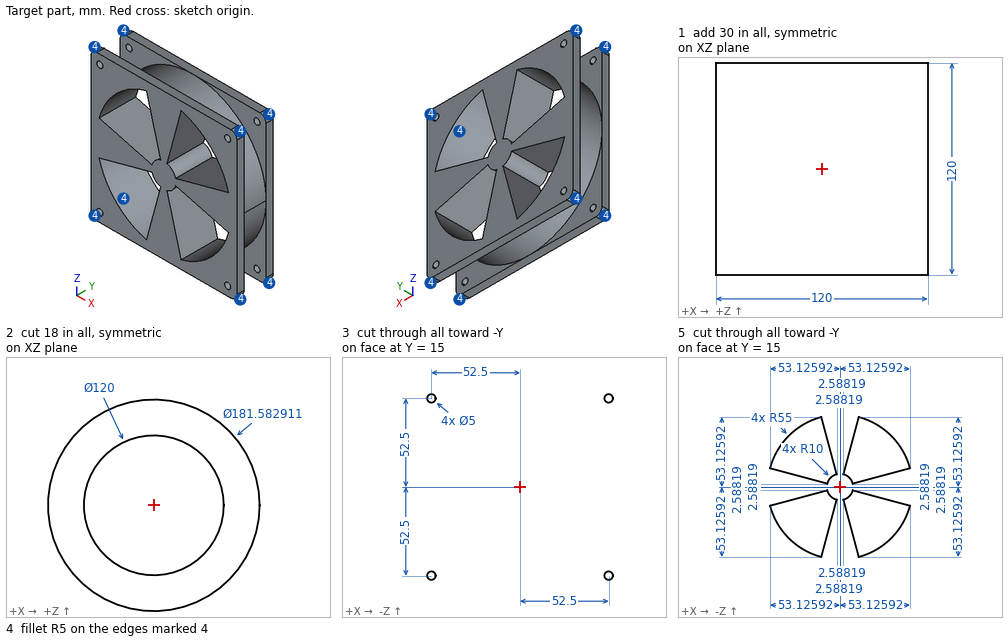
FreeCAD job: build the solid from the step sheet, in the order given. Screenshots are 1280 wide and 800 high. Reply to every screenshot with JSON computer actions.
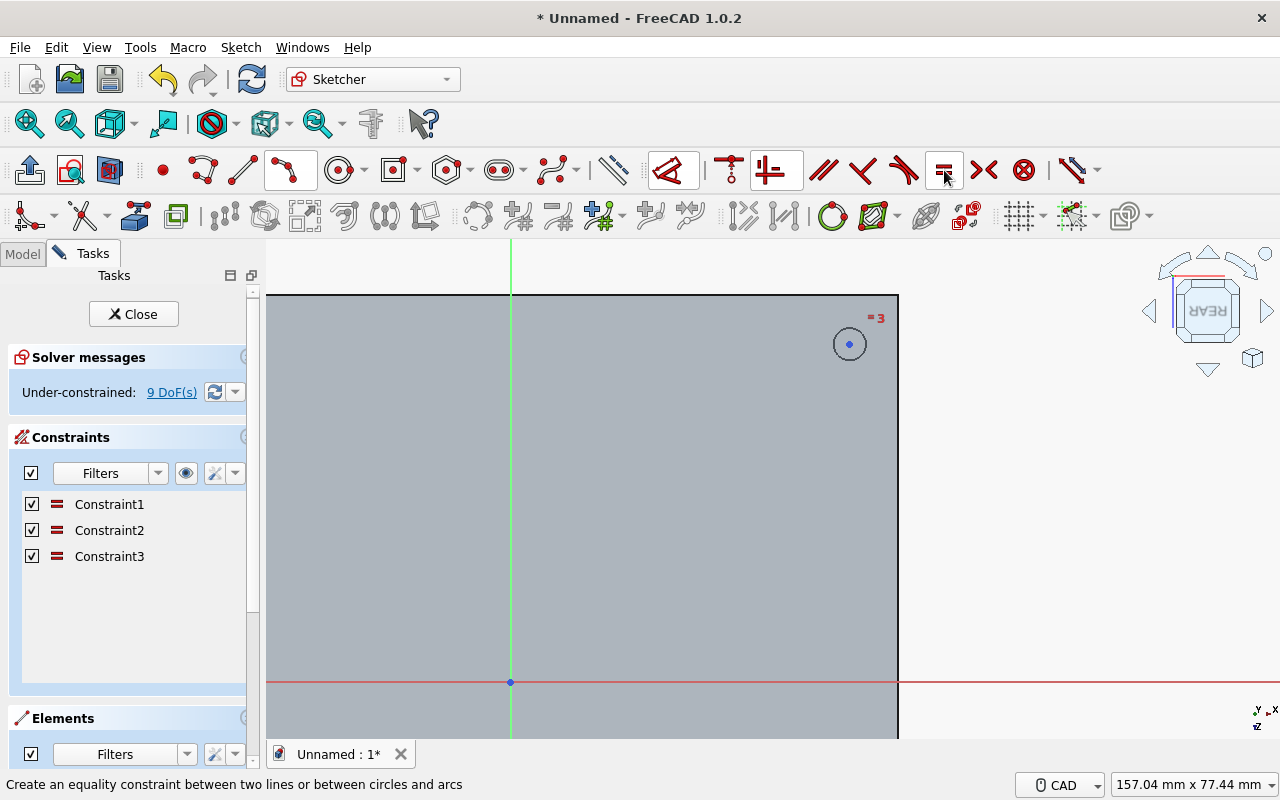
{"action": "scroll", "coordinate": [862, 331], "scroll_direction": "down", "scroll_amount": 4}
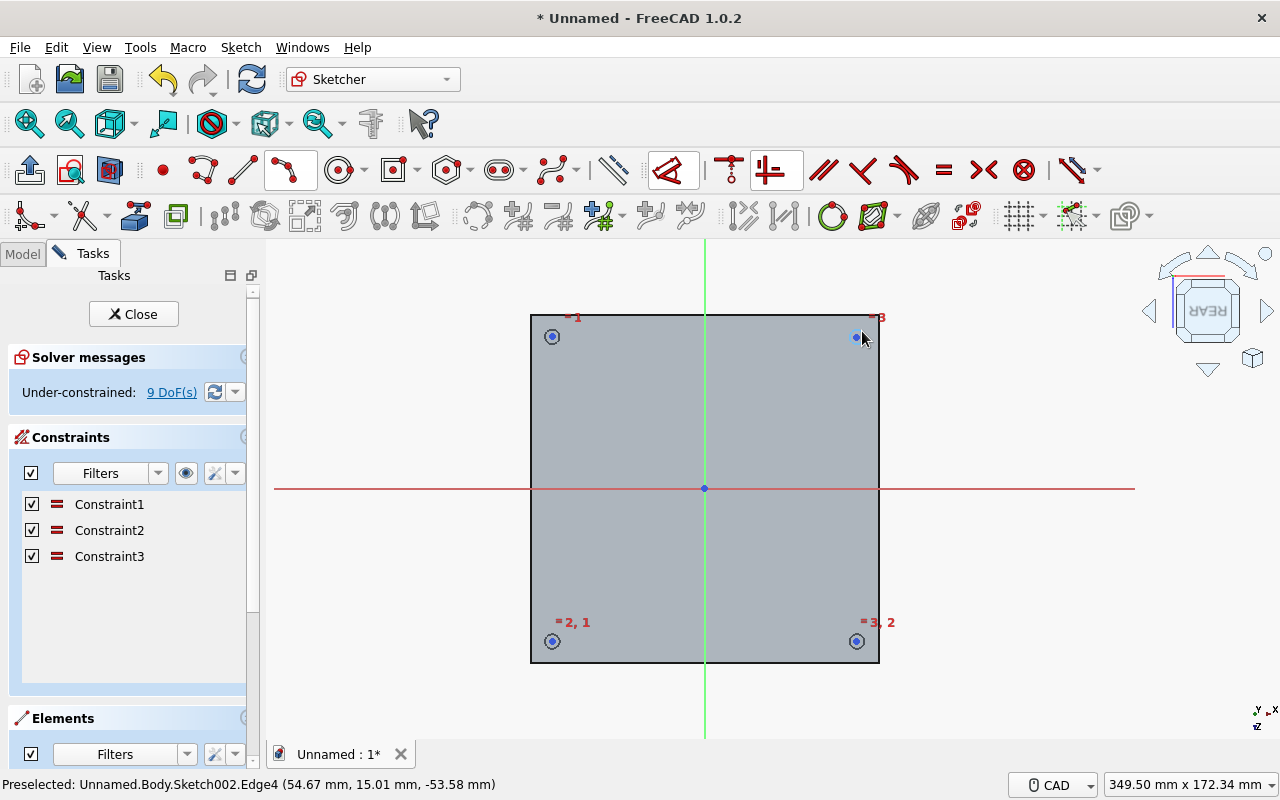
{"action": "left_click", "coordinate": [552, 337]}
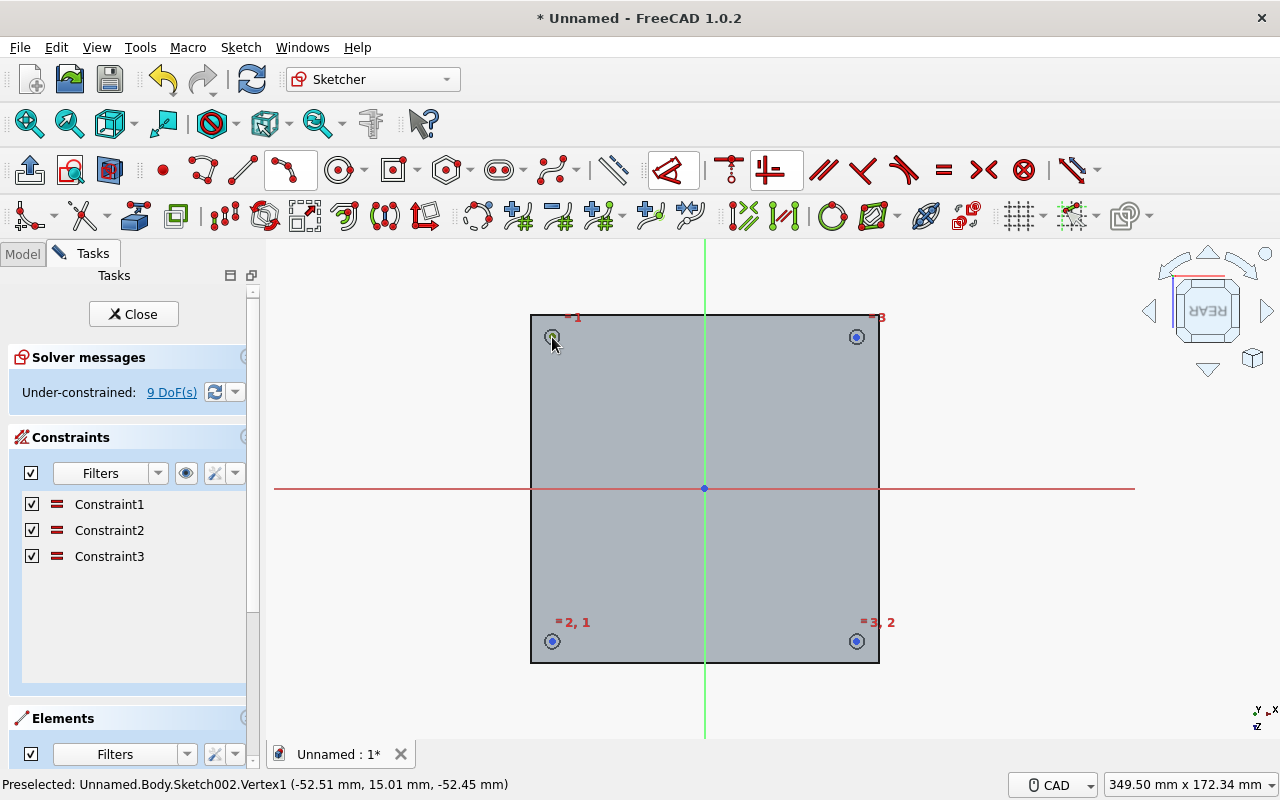
{"action": "left_click", "coordinate": [552, 642]}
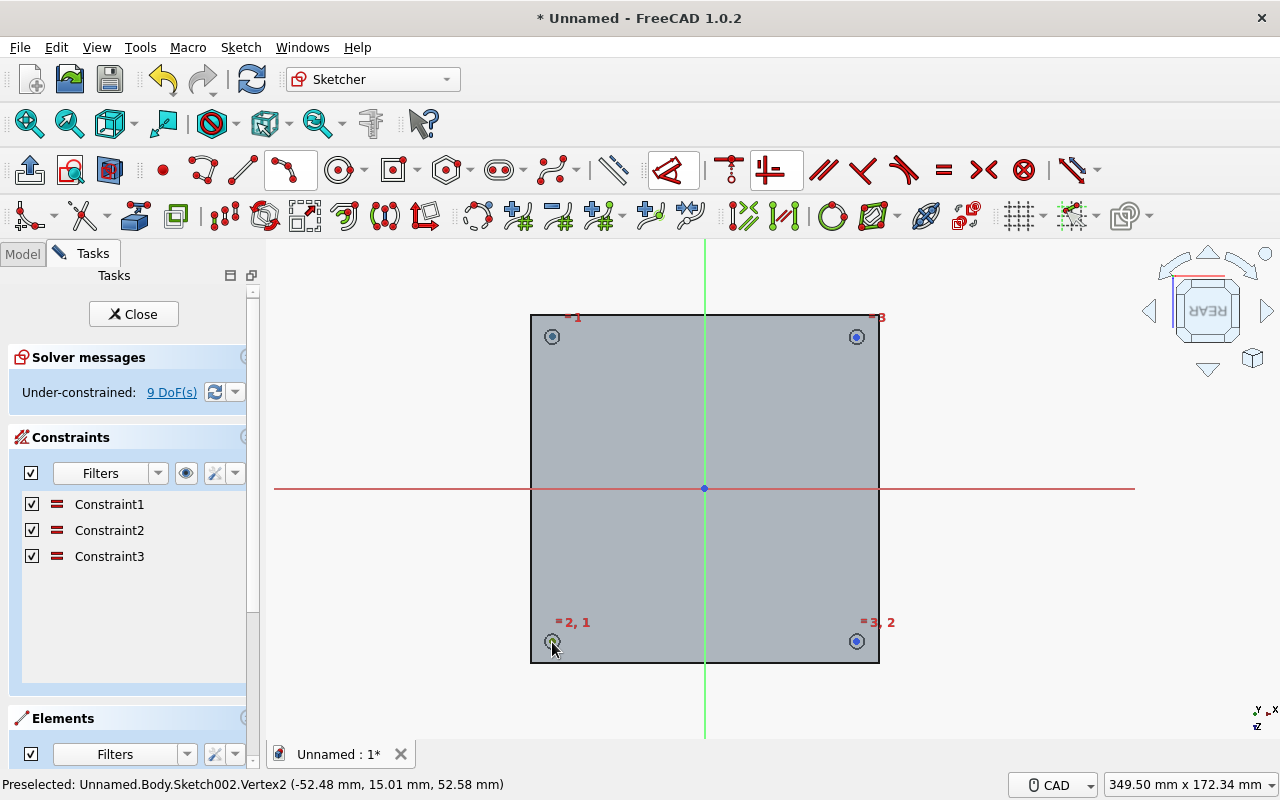
{"action": "key", "text": "v"}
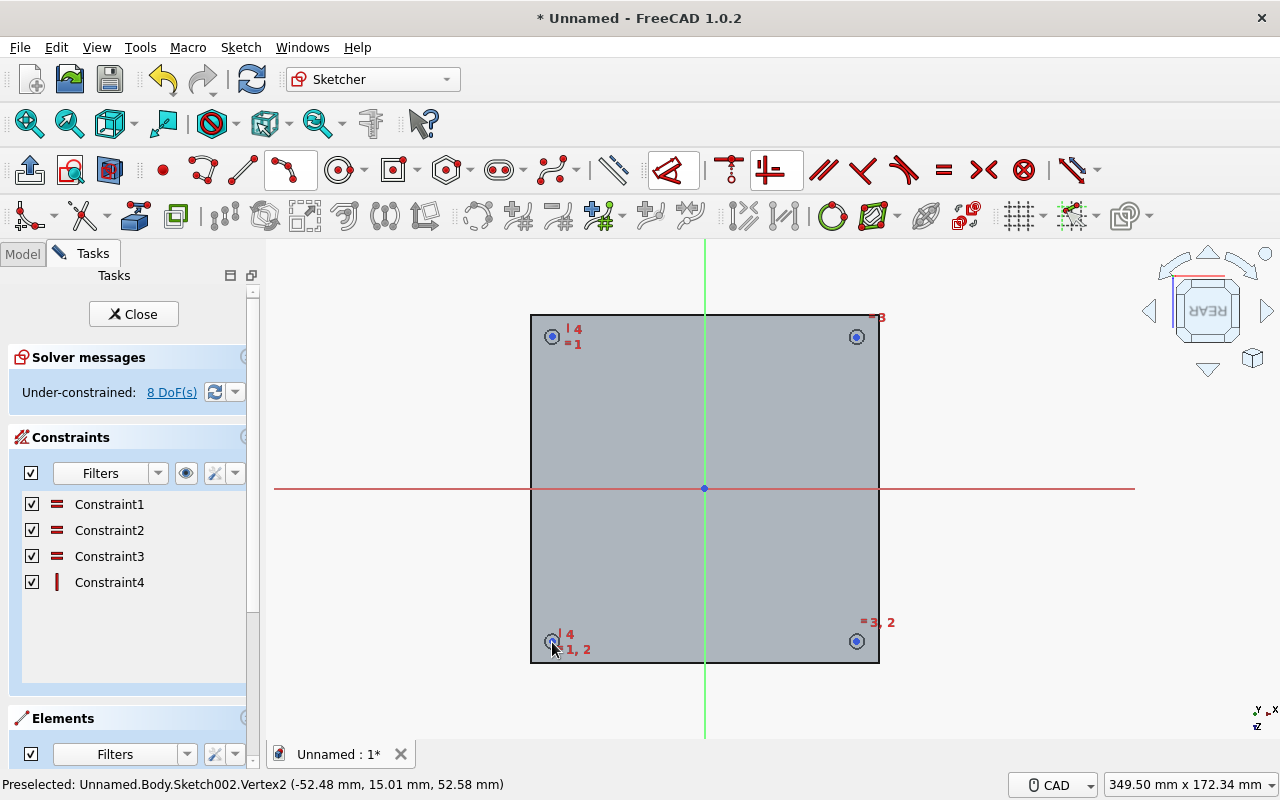
{"action": "left_click", "coordinate": [552, 642]}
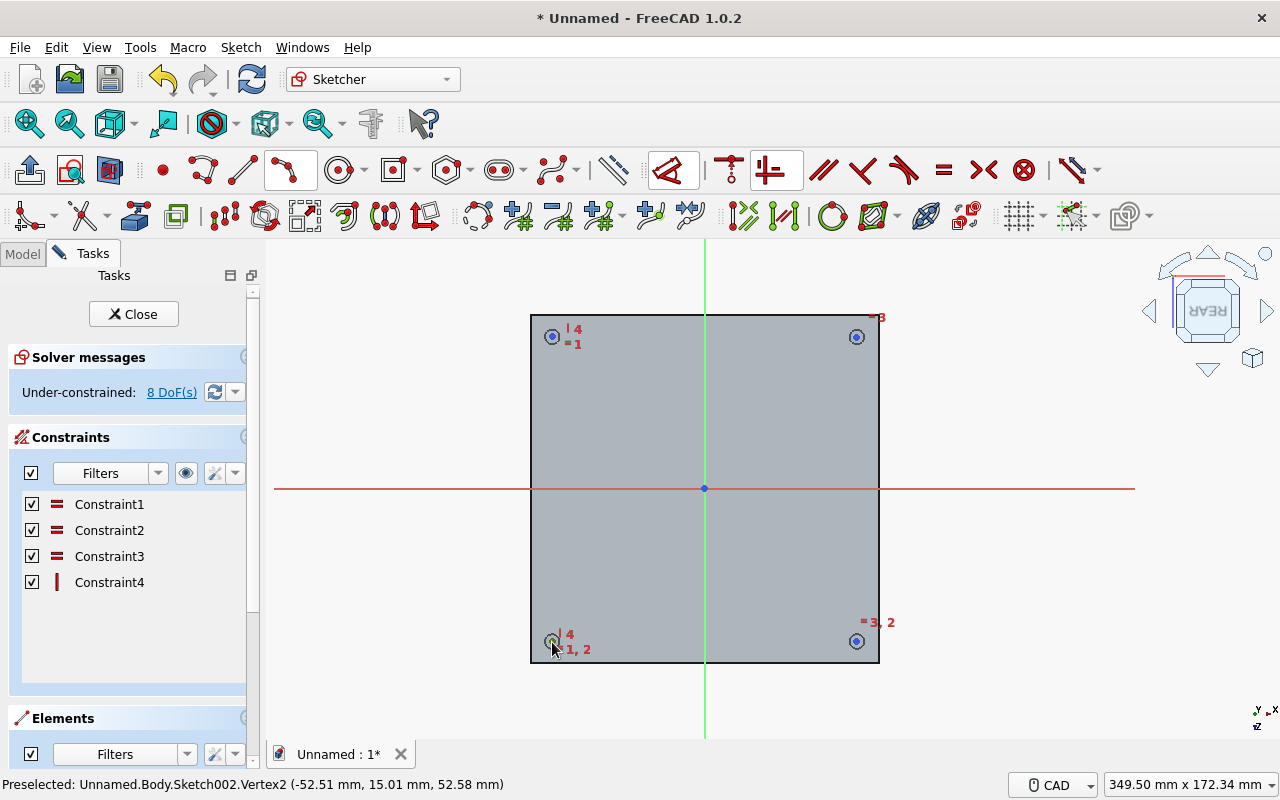
{"action": "left_click", "coordinate": [857, 642]}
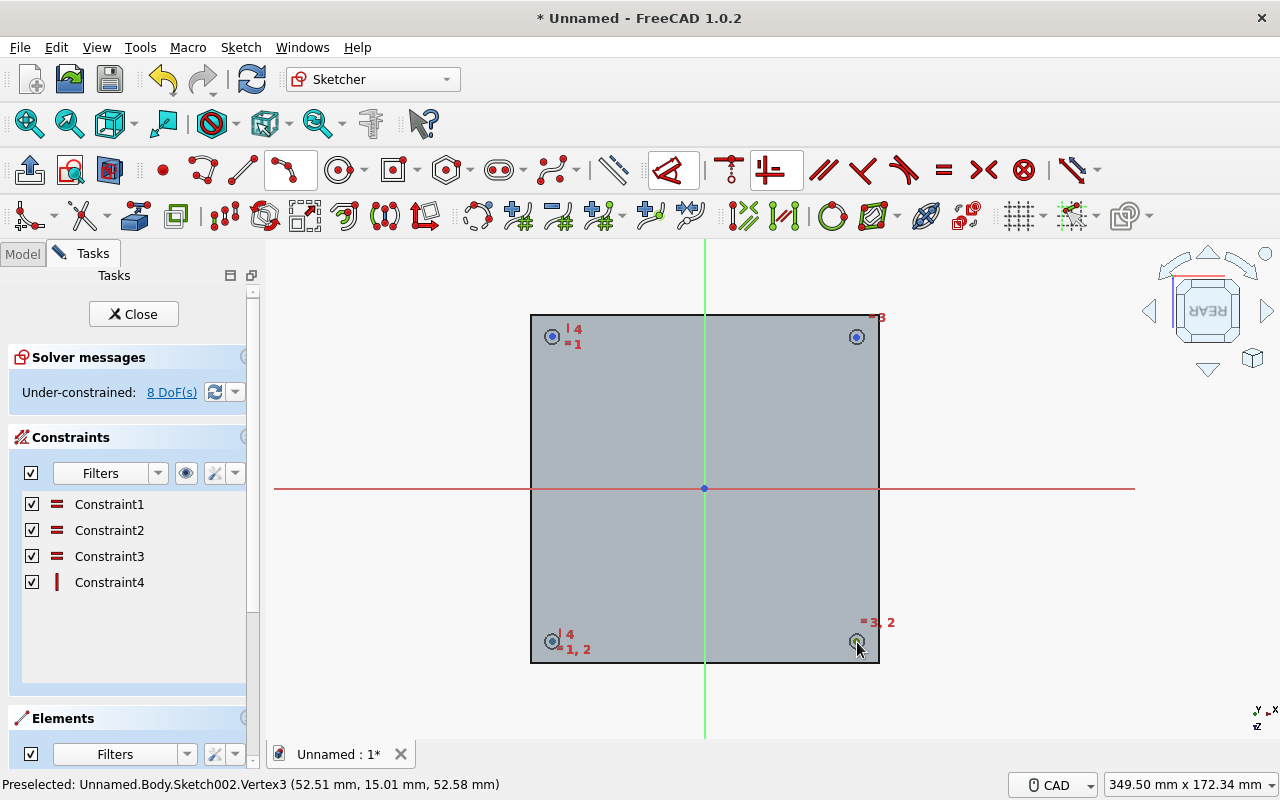
{"action": "left_click", "coordinate": [798, 170]}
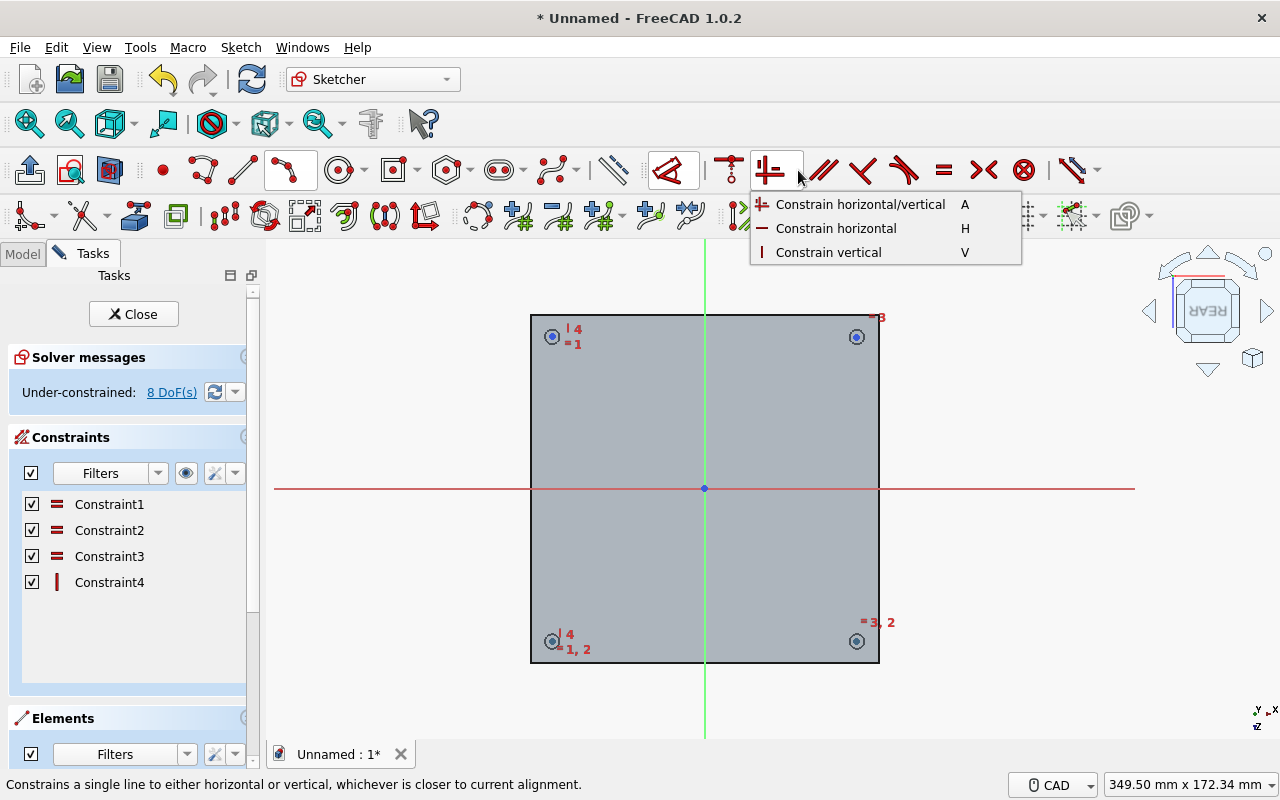
{"action": "left_click", "coordinate": [886, 228]}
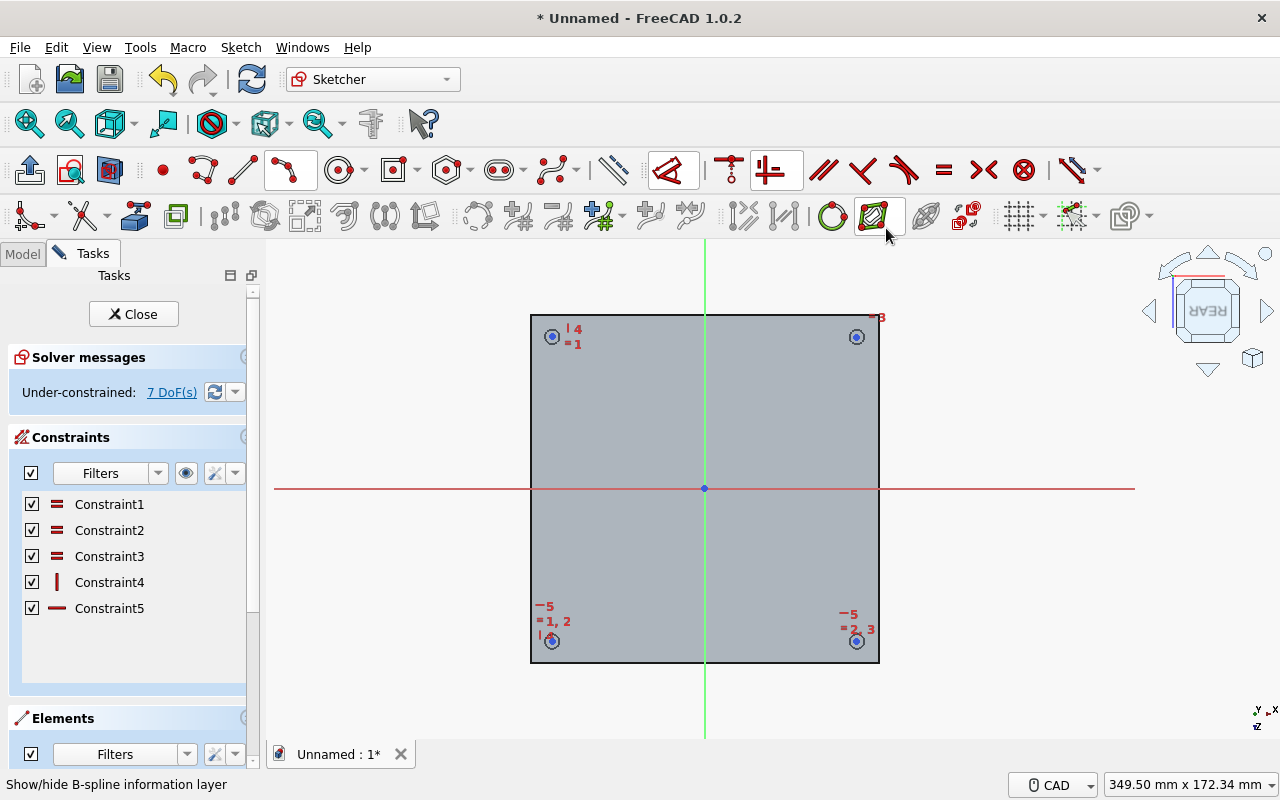
{"action": "left_click", "coordinate": [857, 642]}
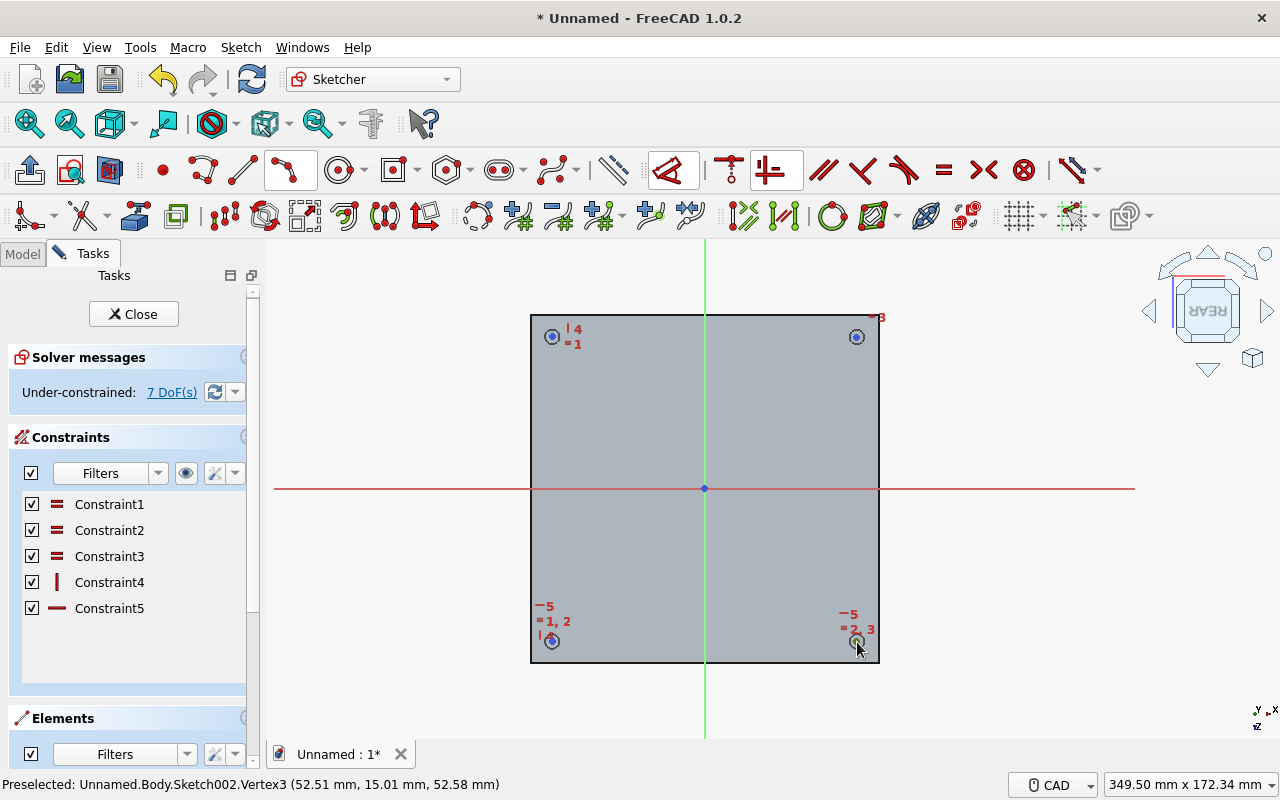
{"action": "left_click", "coordinate": [857, 337]}